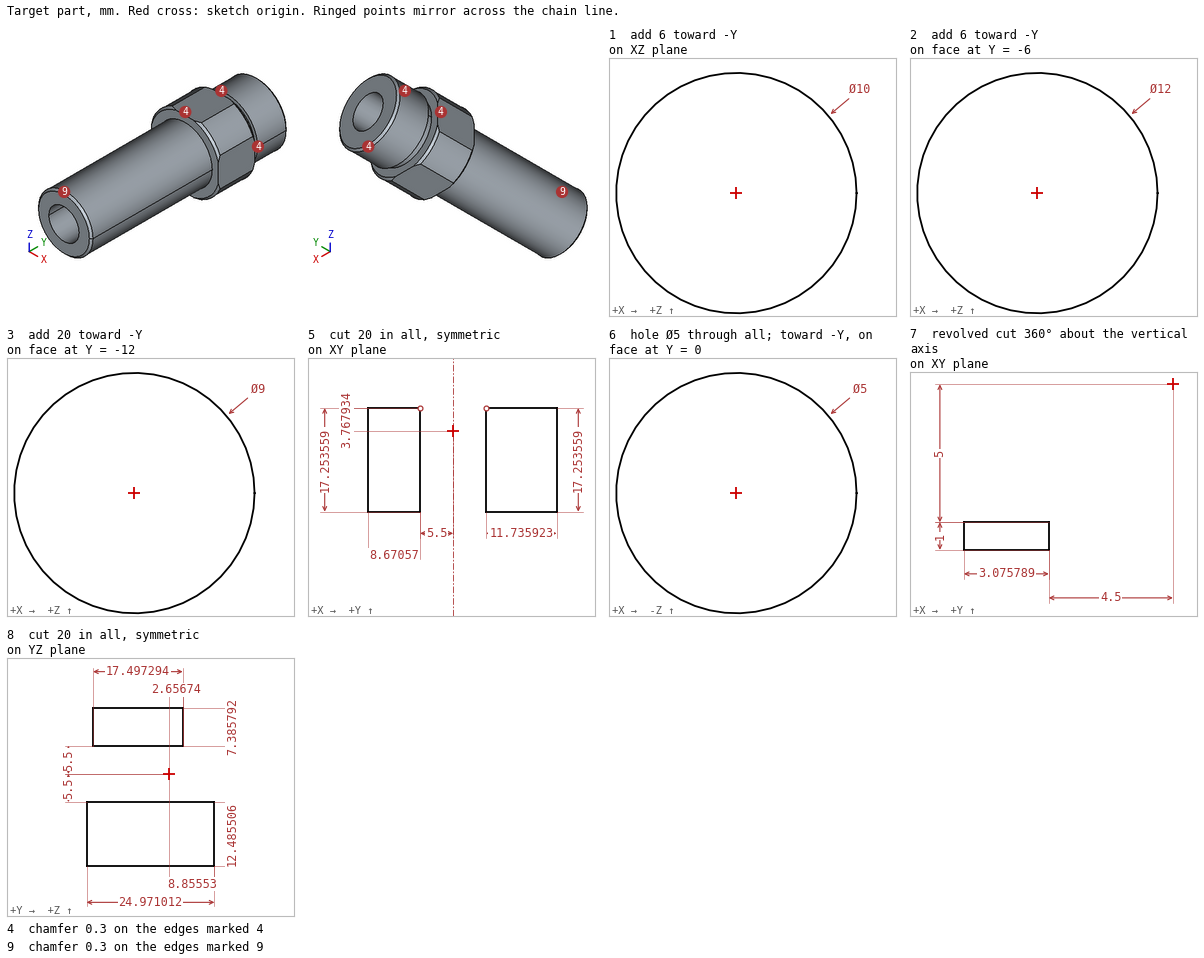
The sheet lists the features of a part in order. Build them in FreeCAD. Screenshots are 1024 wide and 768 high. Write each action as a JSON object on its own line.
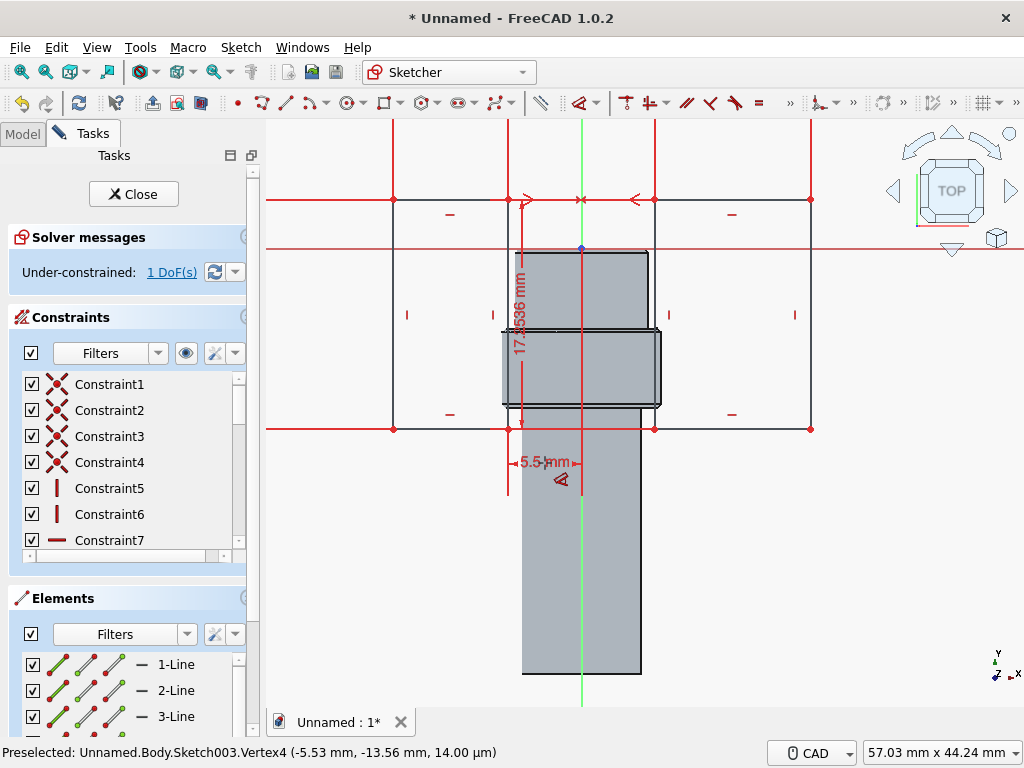
{"action": "left_click", "coordinate": [393, 200]}
{"action": "left_click", "coordinate": [359, 224]}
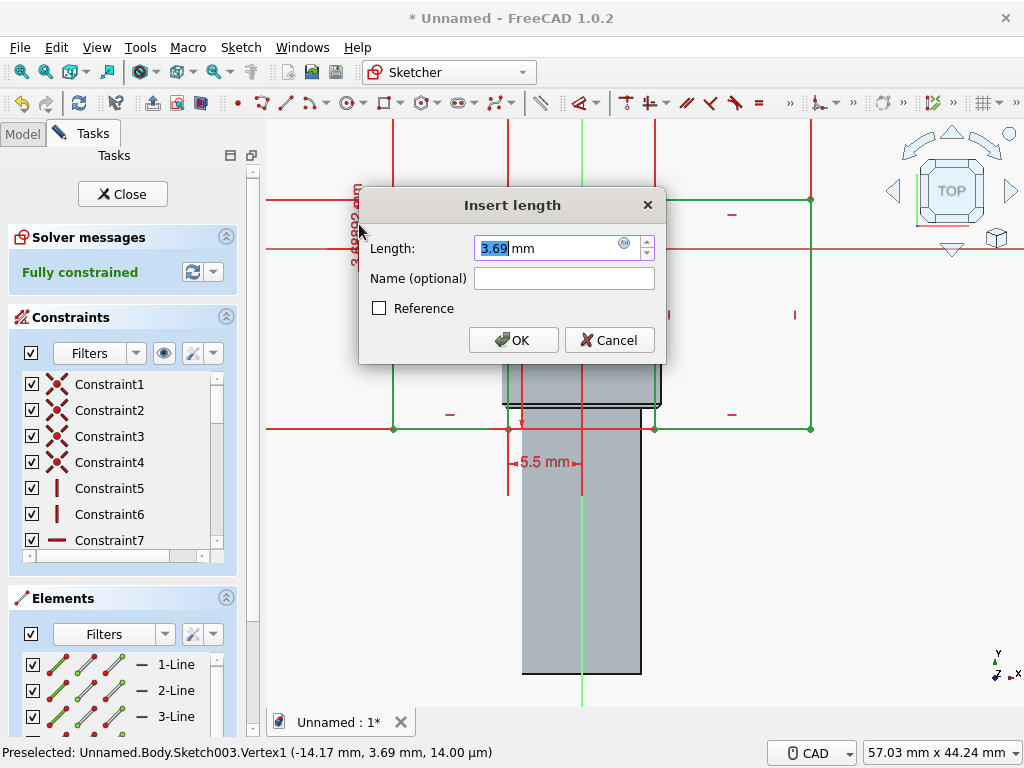
{"action": "type", "text": "3.767934"}
{"action": "key", "text": "Return"}
{"action": "key", "text": "Escape"}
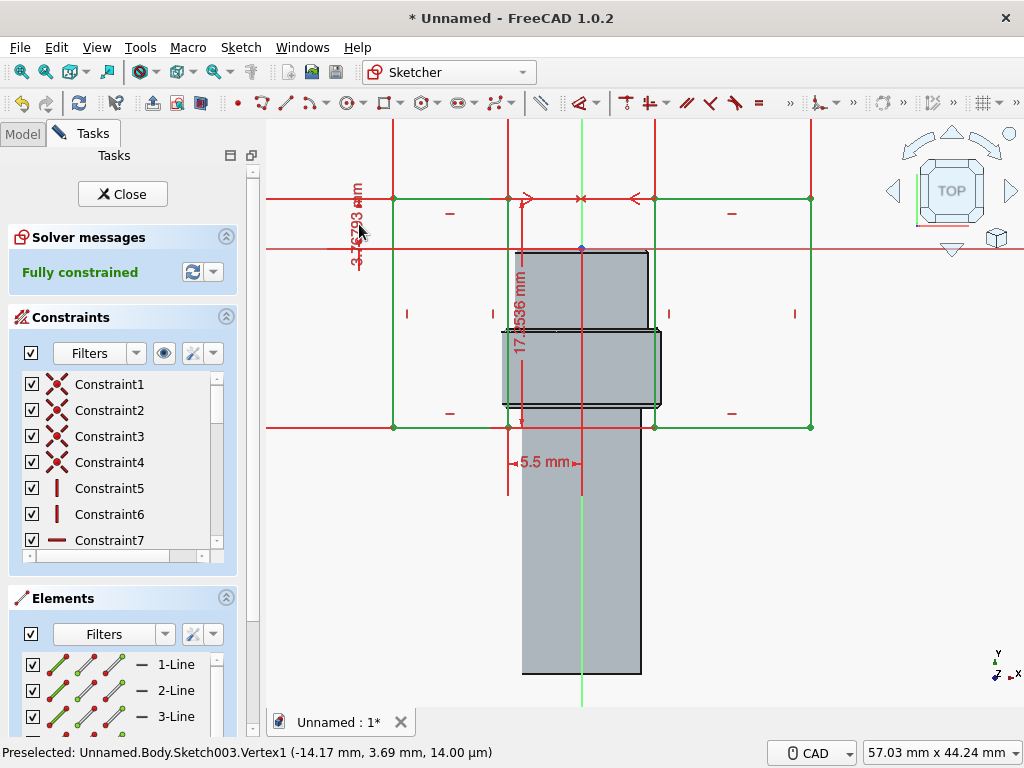
{"action": "left_click", "coordinate": [123, 194]}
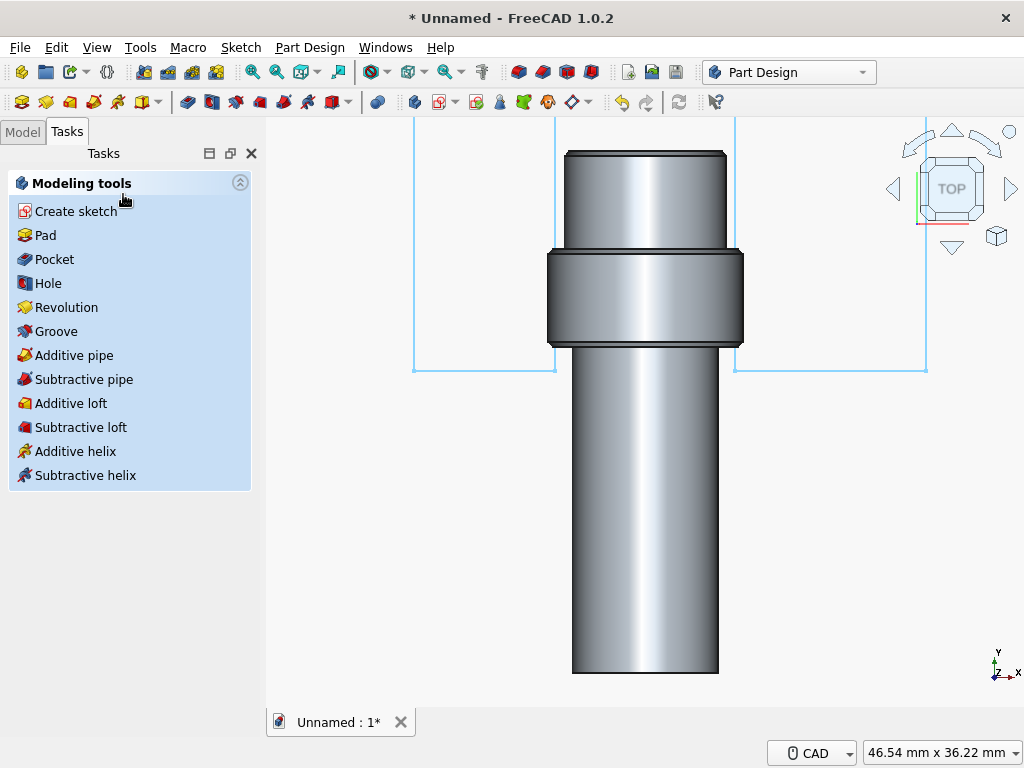
{"action": "left_click", "coordinate": [188, 102]}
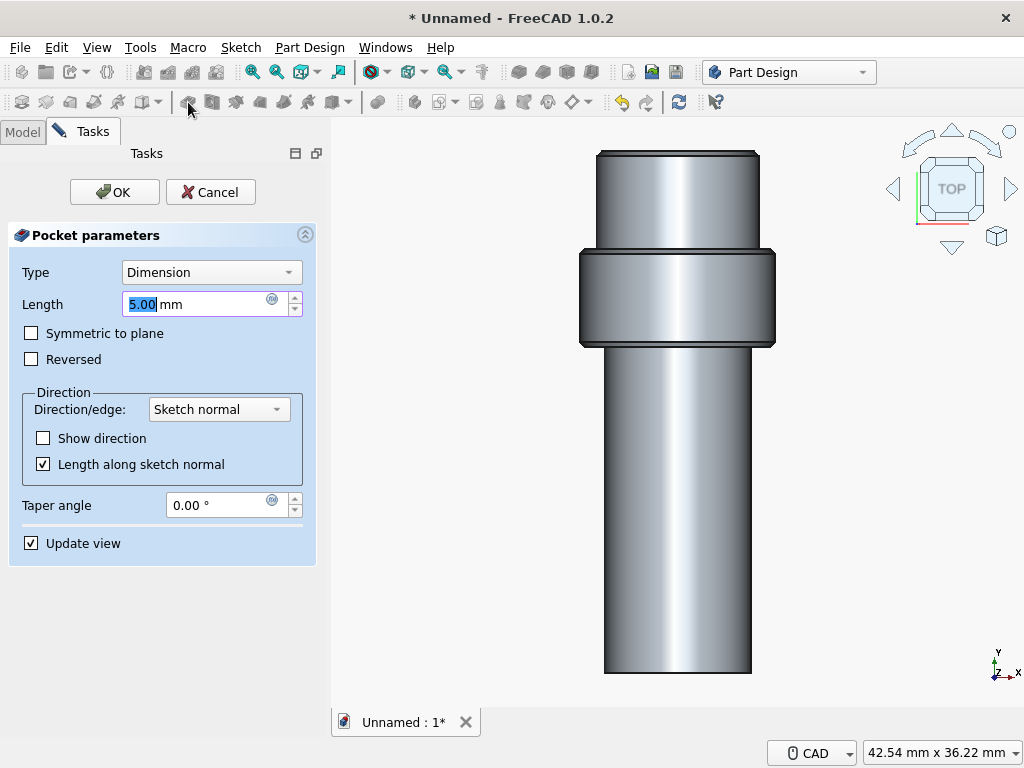
{"action": "type", "text": "20"}
{"action": "key", "text": "Tab"}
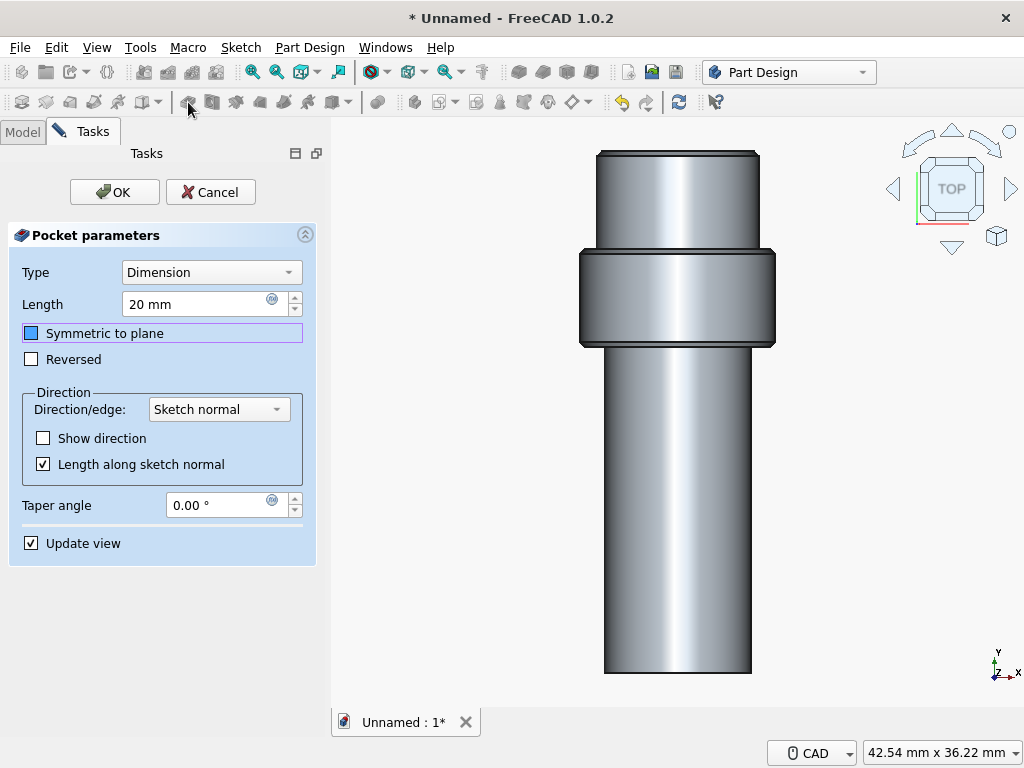
{"action": "left_click", "coordinate": [30, 333]}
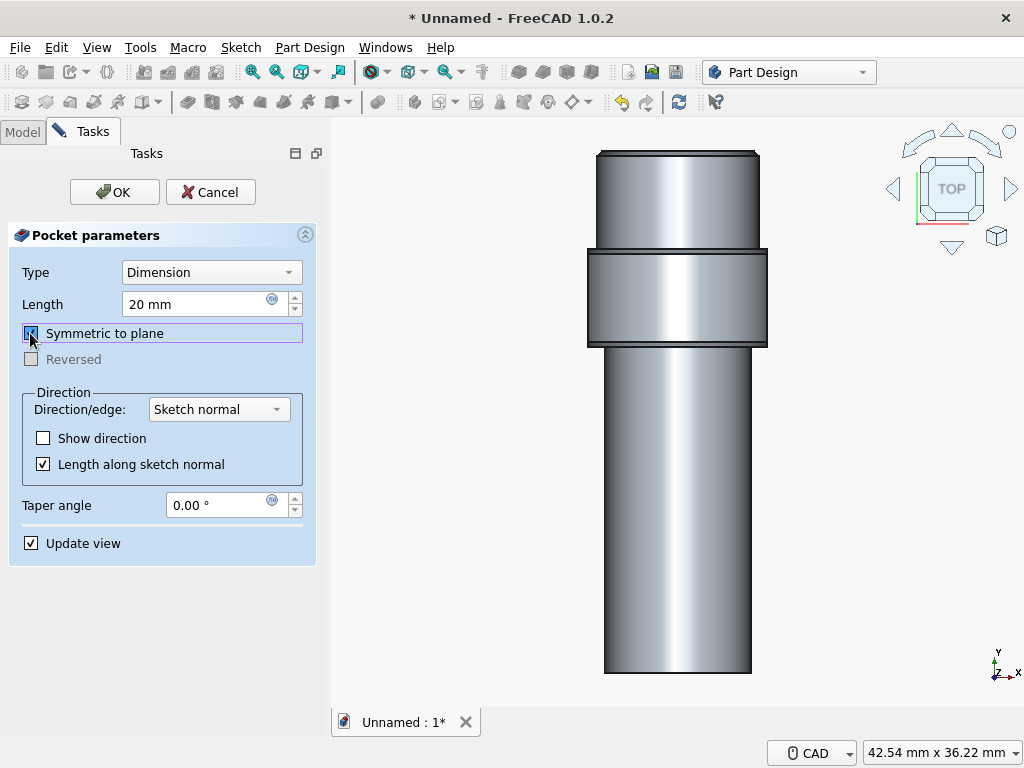
{"action": "left_click", "coordinate": [115, 192]}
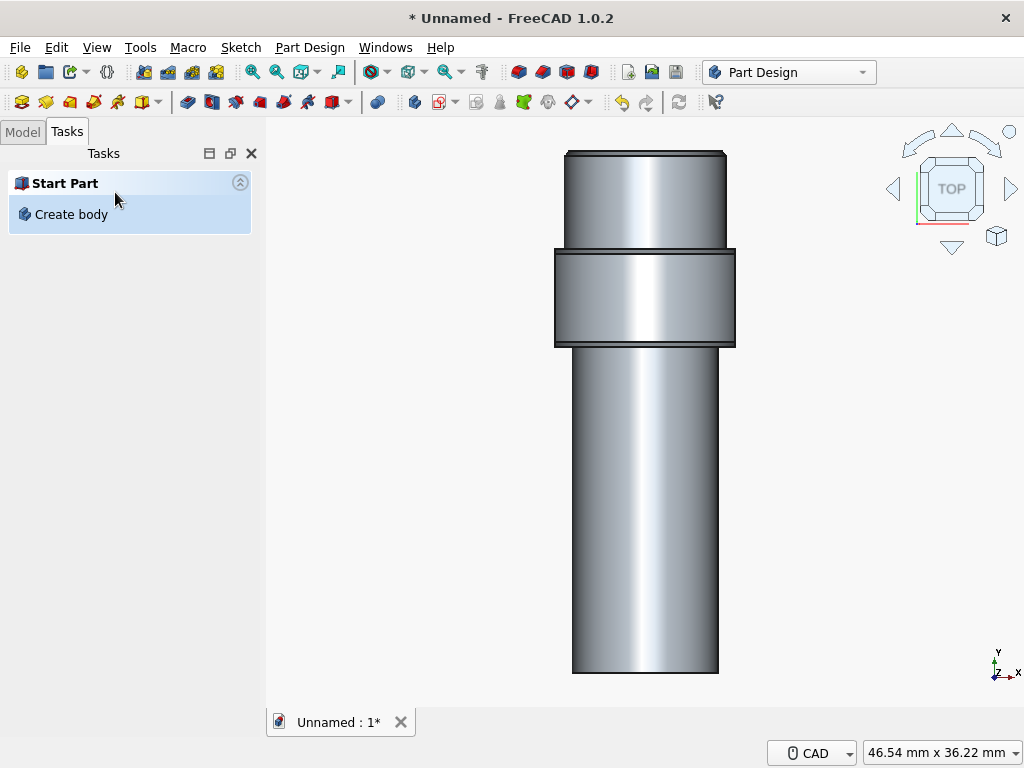
{"action": "key", "text": "4"}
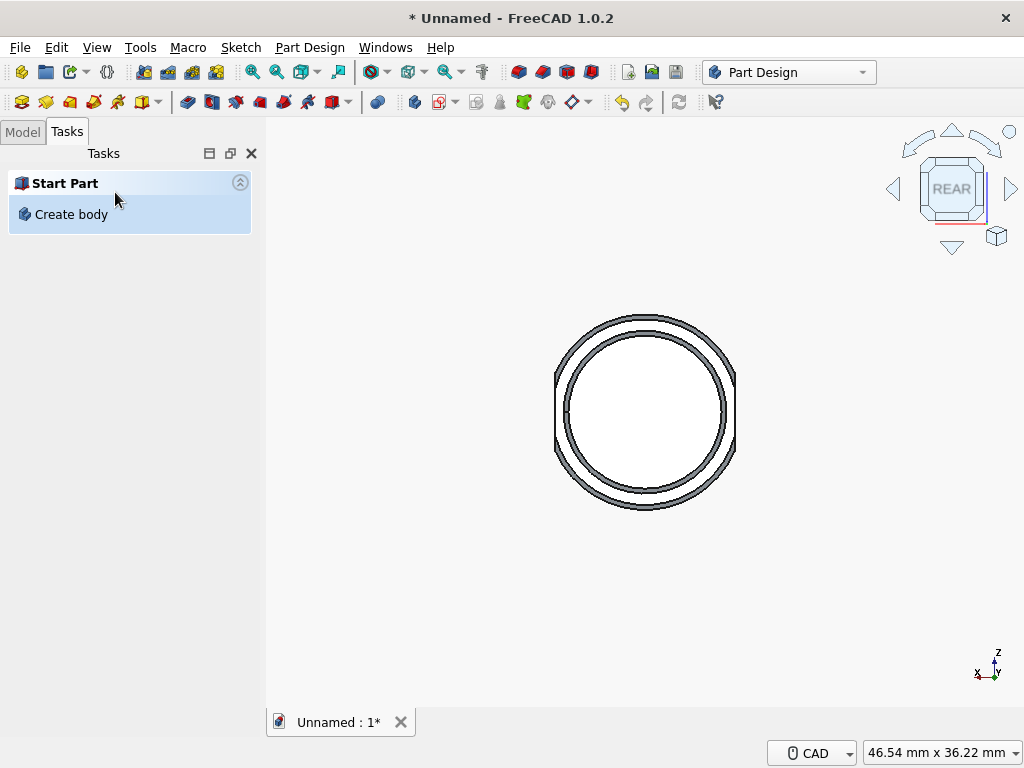
{"action": "key", "text": "v f"}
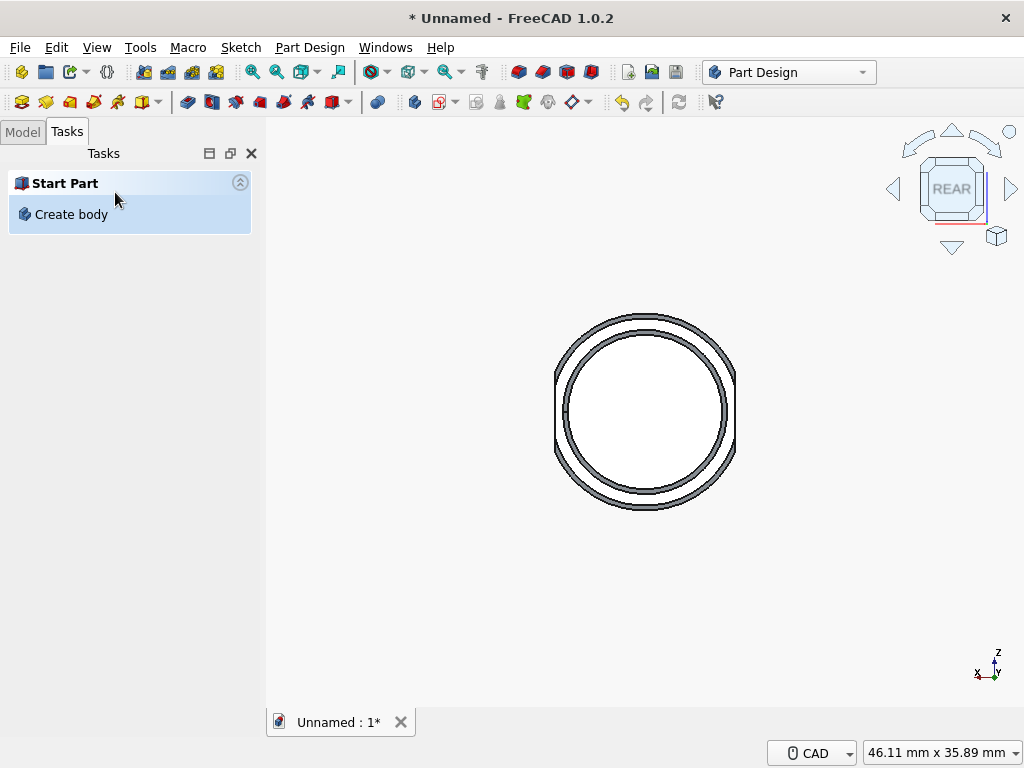
{"action": "left_click", "coordinate": [645, 411]}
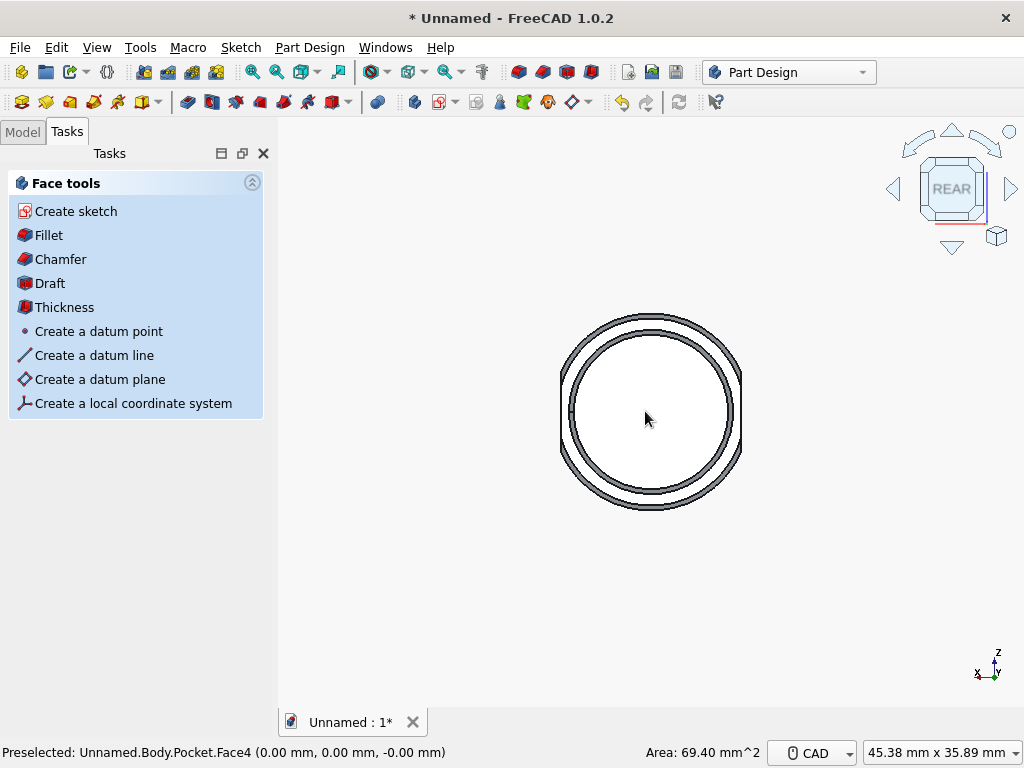
{"action": "left_click", "coordinate": [440, 102]}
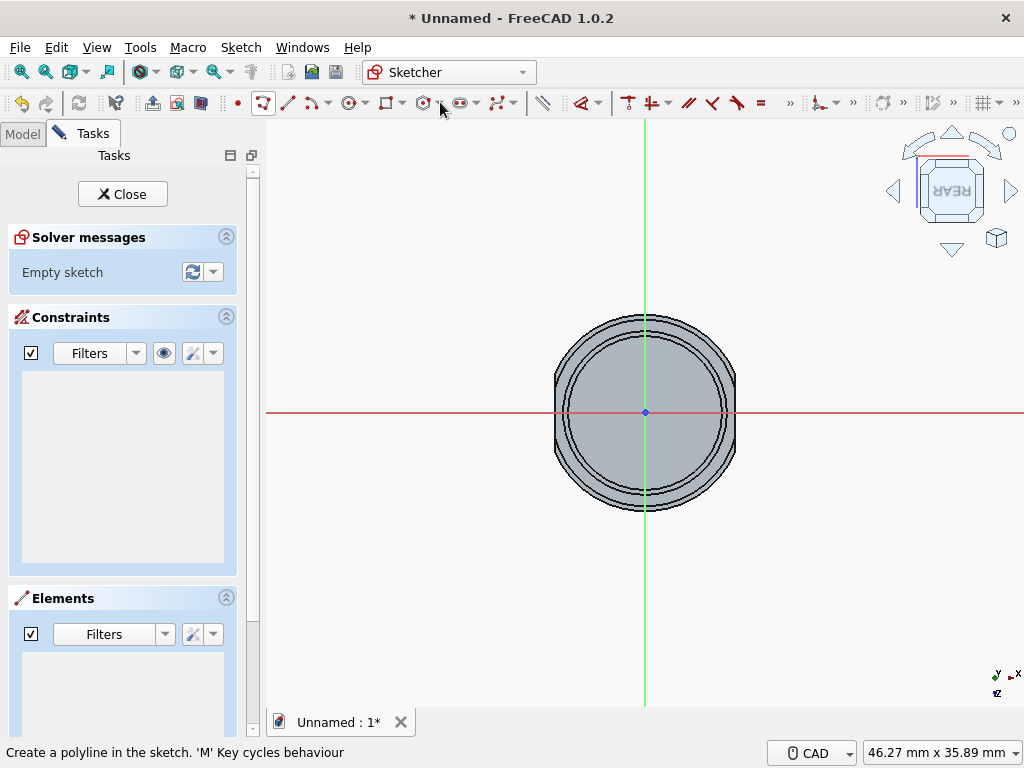
{"action": "scroll", "coordinate": [662, 413], "scroll_direction": "up", "scroll_amount": 8}